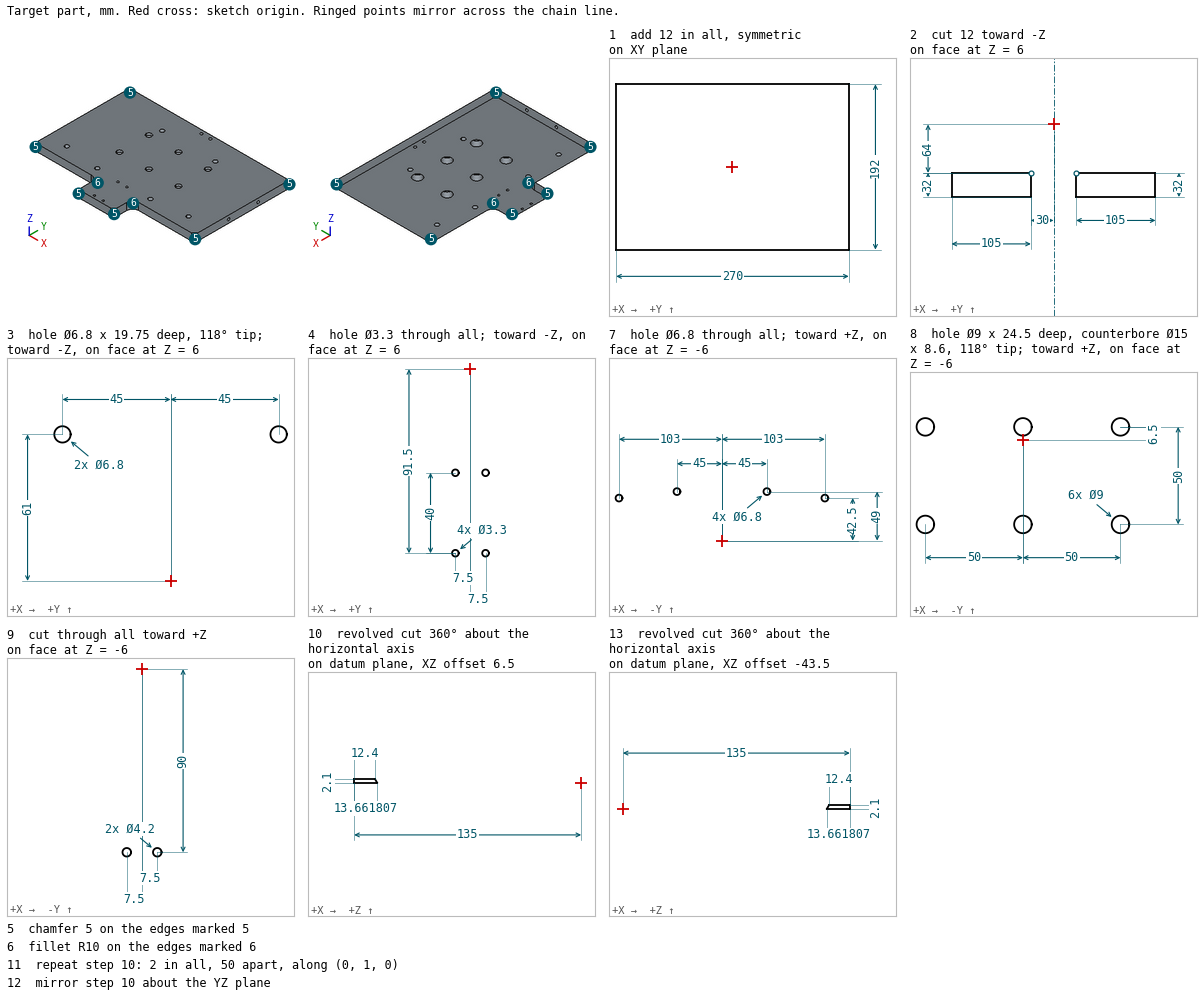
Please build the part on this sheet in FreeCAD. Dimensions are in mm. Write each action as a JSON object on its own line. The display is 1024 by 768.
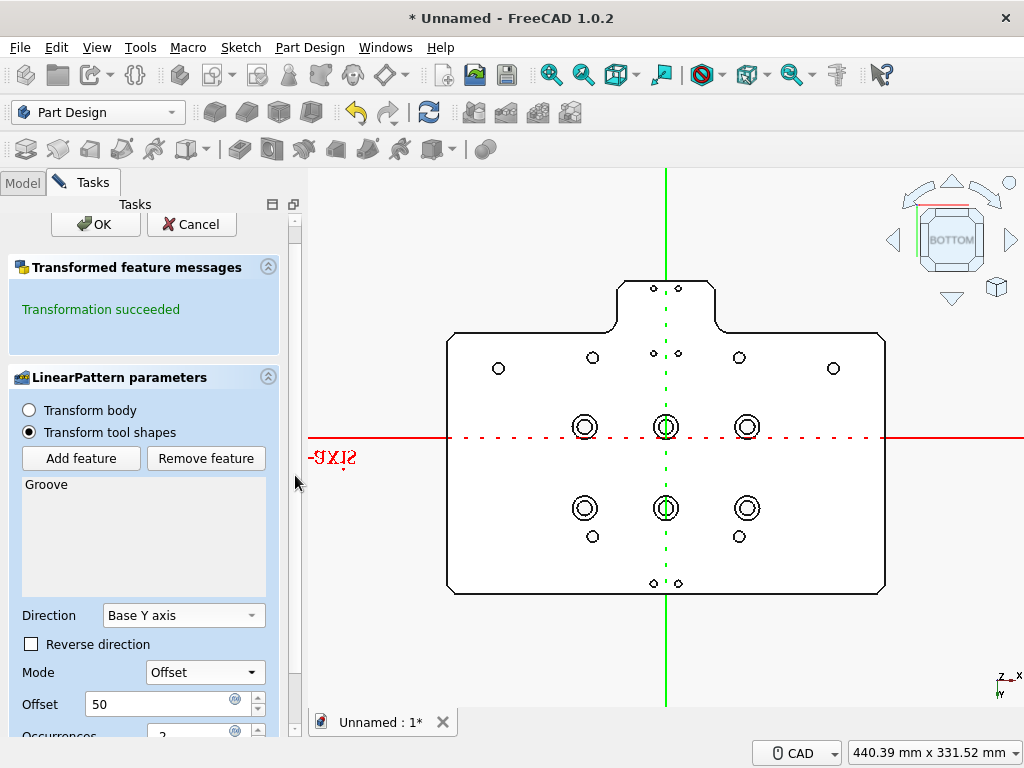
{"action": "left_click", "coordinate": [96, 243]}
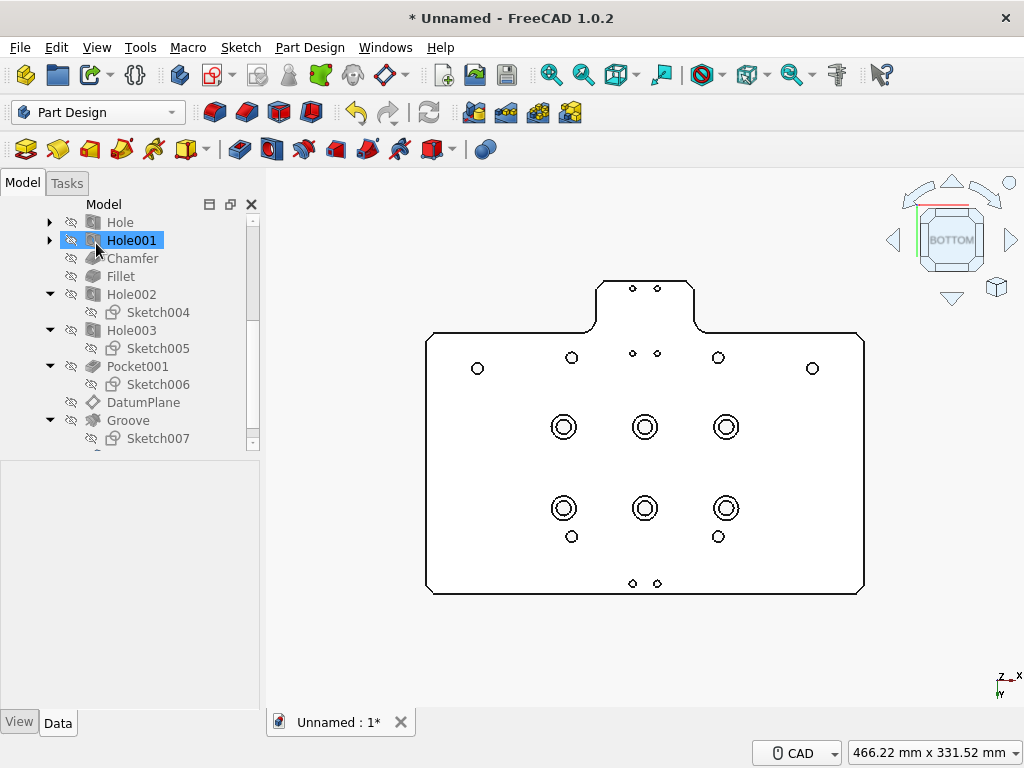
{"action": "left_click", "coordinate": [116, 420]}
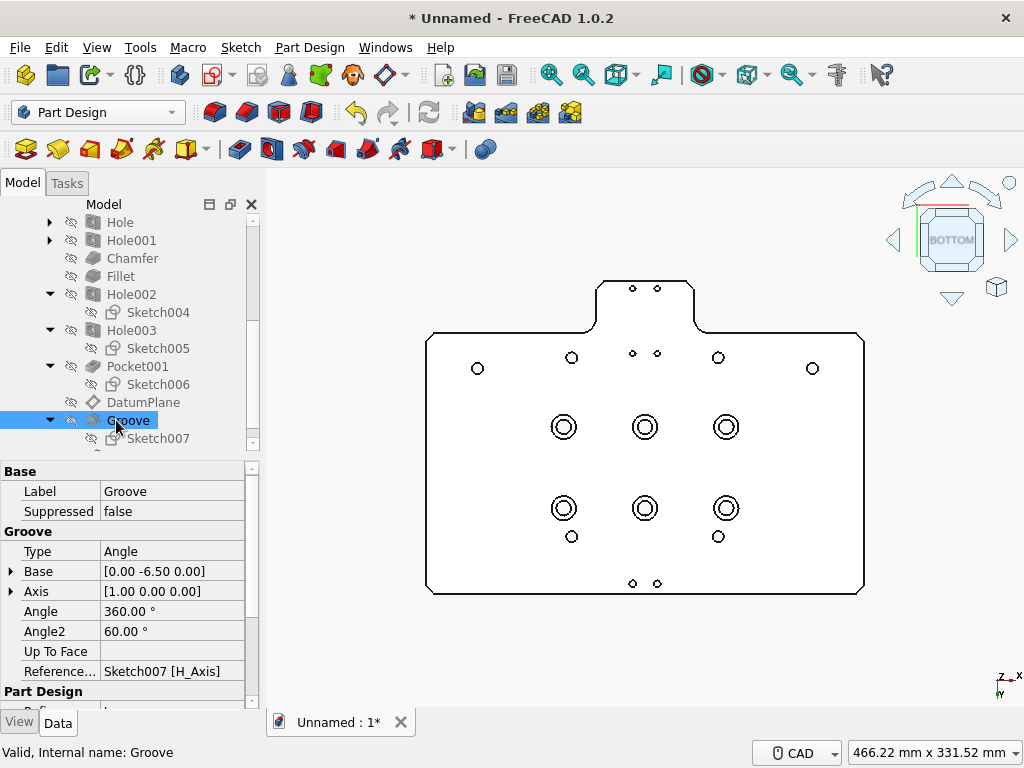
{"action": "left_click", "coordinate": [474, 112]}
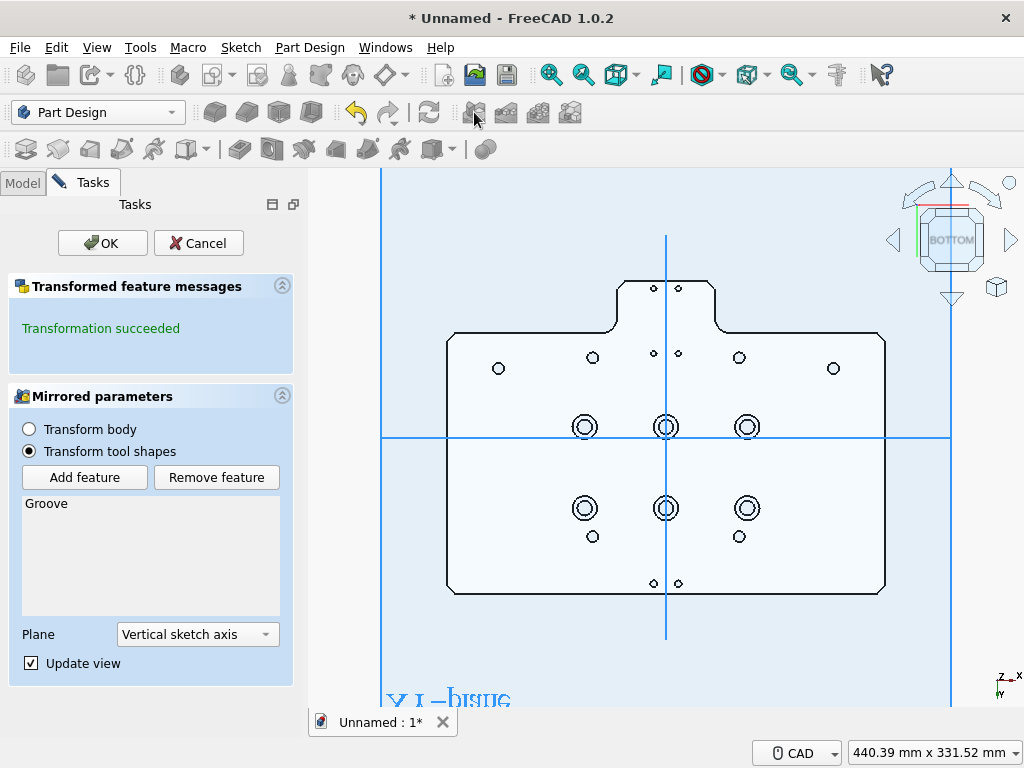
{"action": "left_click", "coordinate": [198, 634]}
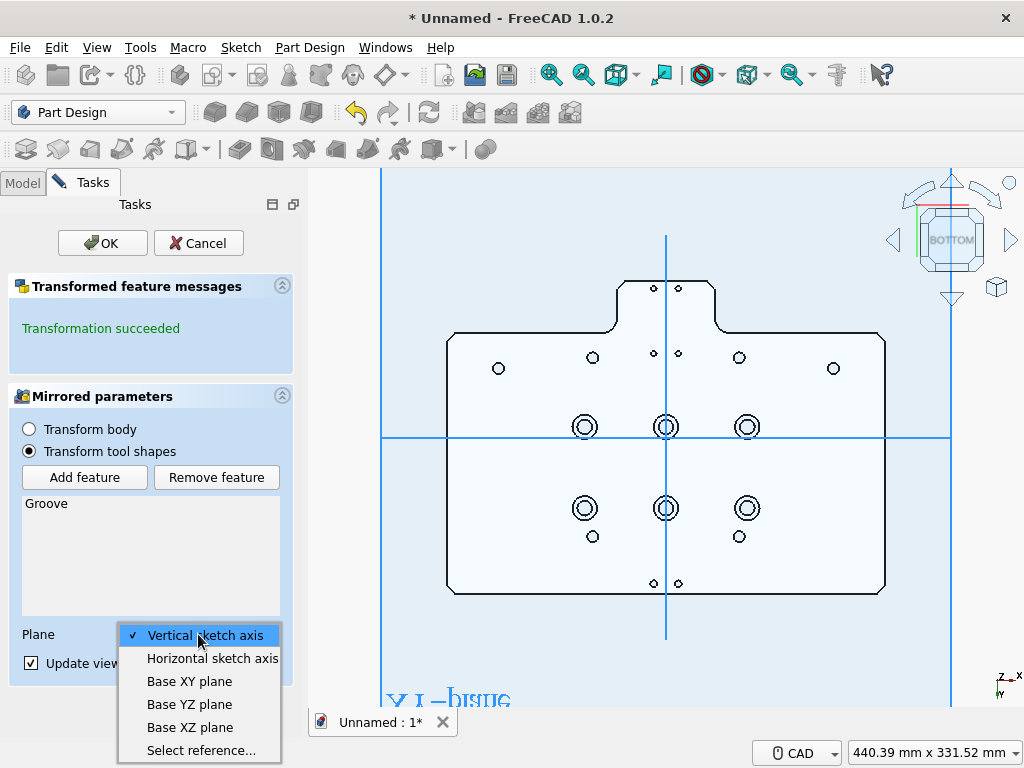
{"action": "left_click", "coordinate": [198, 704]}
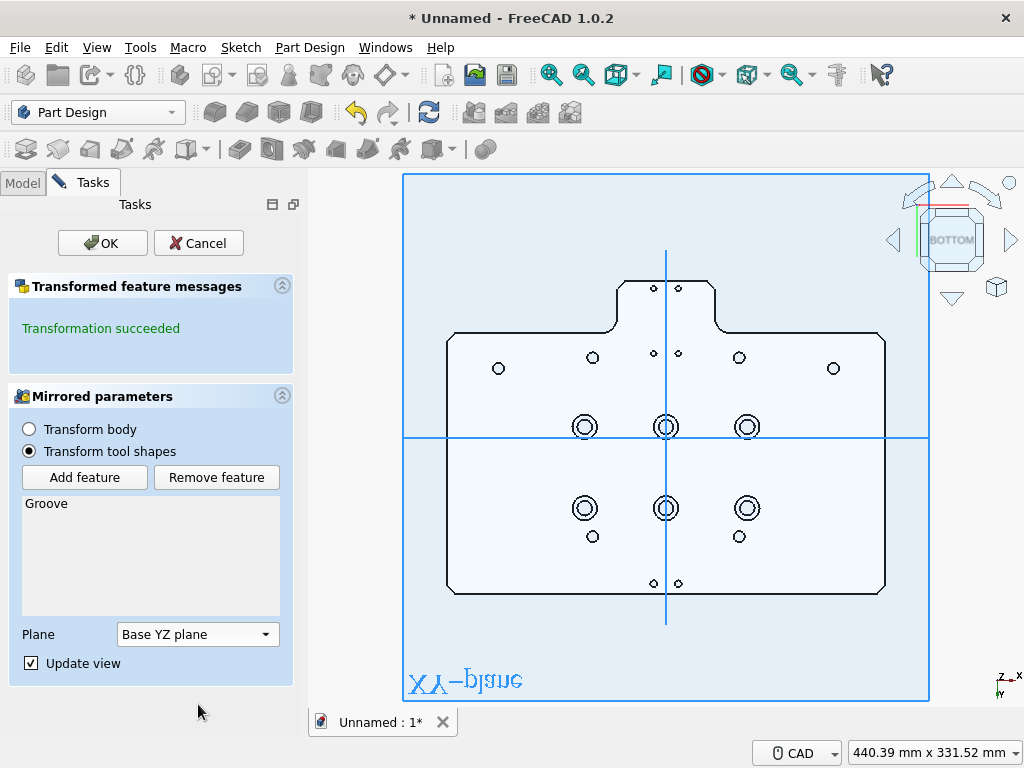
{"action": "left_click", "coordinate": [103, 243]}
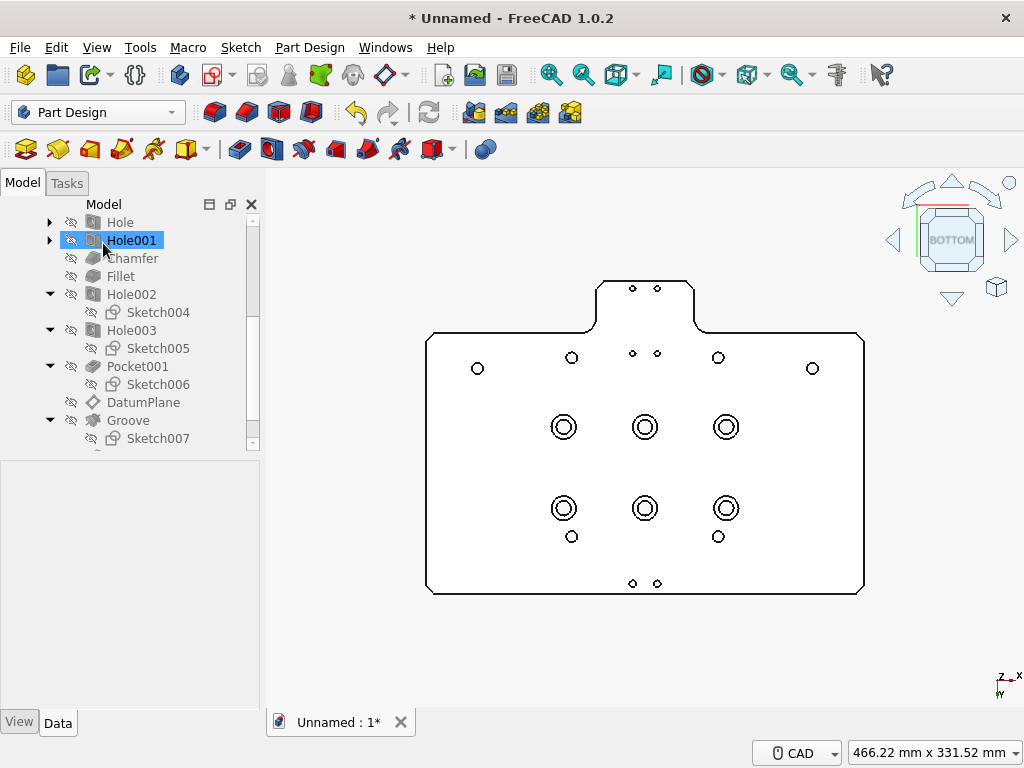
{"action": "scroll", "coordinate": [140, 326], "scroll_direction": "down", "scroll_amount": 3}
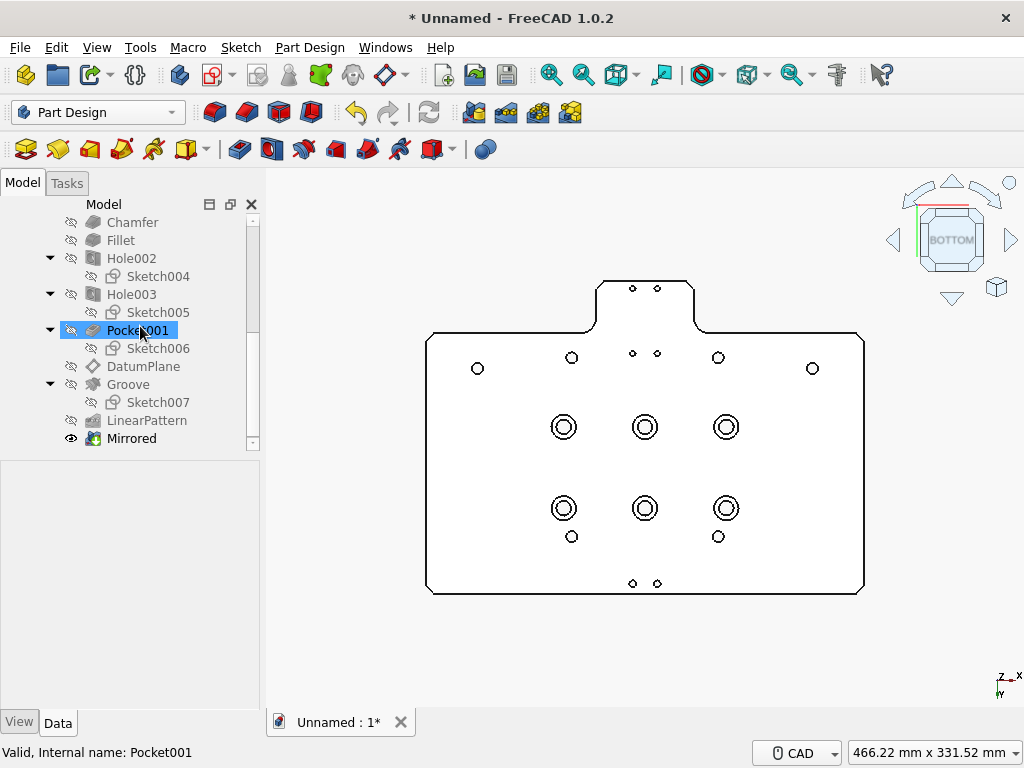
{"action": "scroll", "coordinate": [140, 326], "scroll_direction": "up", "scroll_amount": 15}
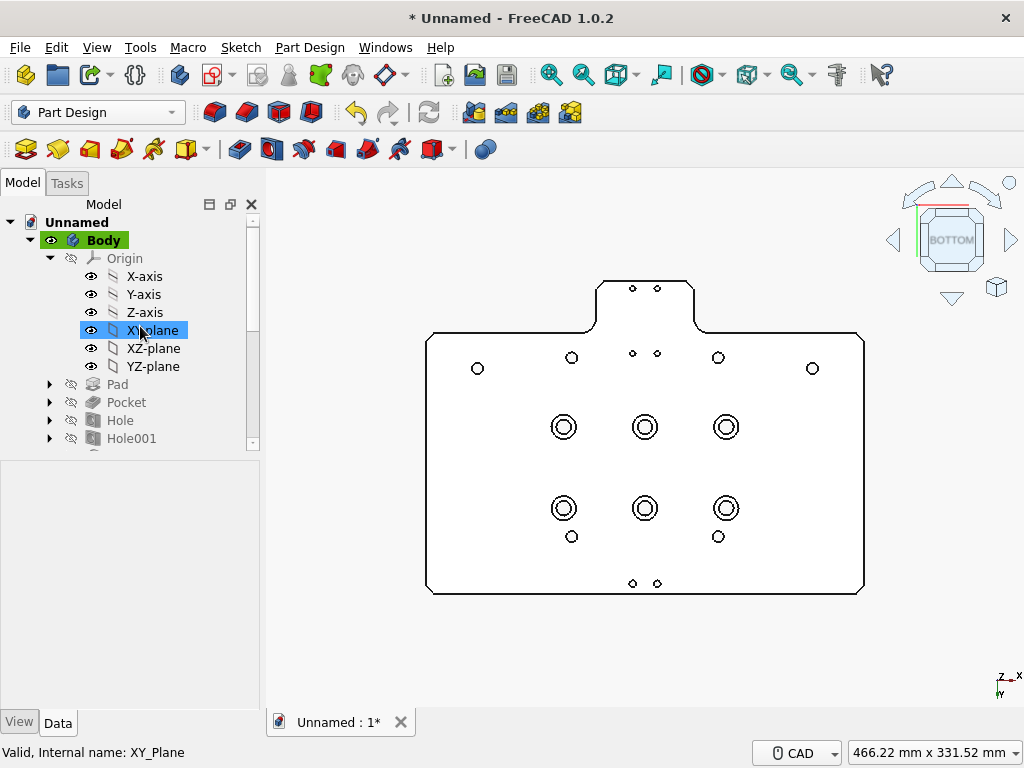
{"action": "left_click", "coordinate": [136, 348]}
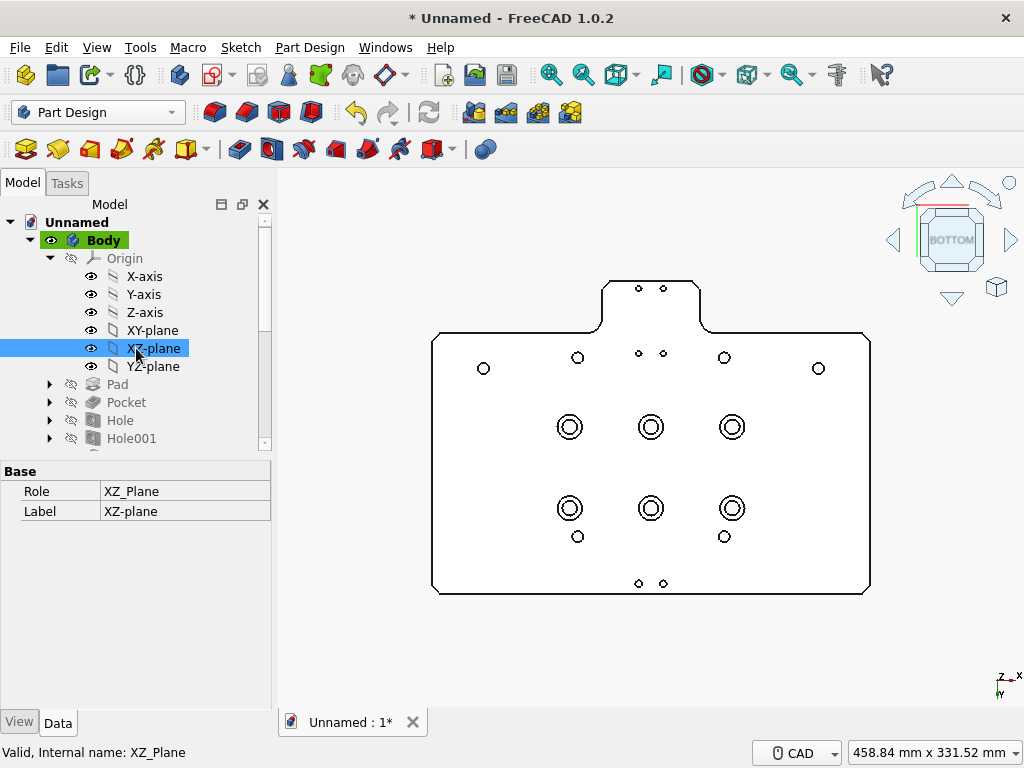
{"action": "left_click", "coordinate": [386, 76]}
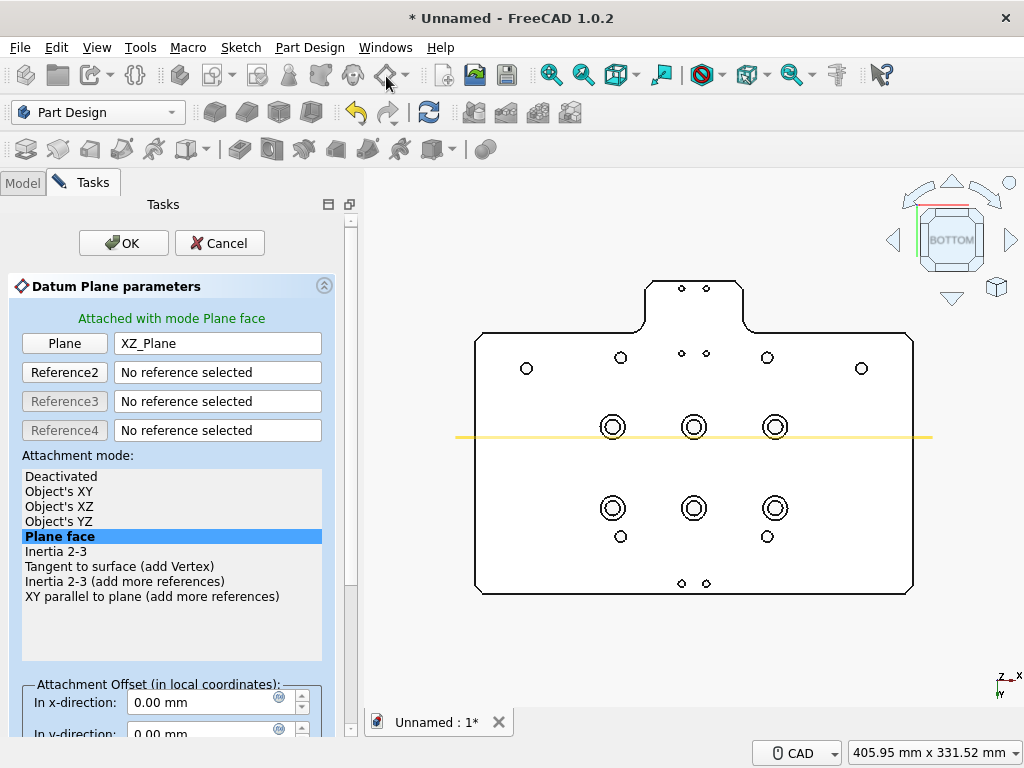
{"action": "scroll", "coordinate": [351, 475], "scroll_direction": "down", "scroll_amount": 2}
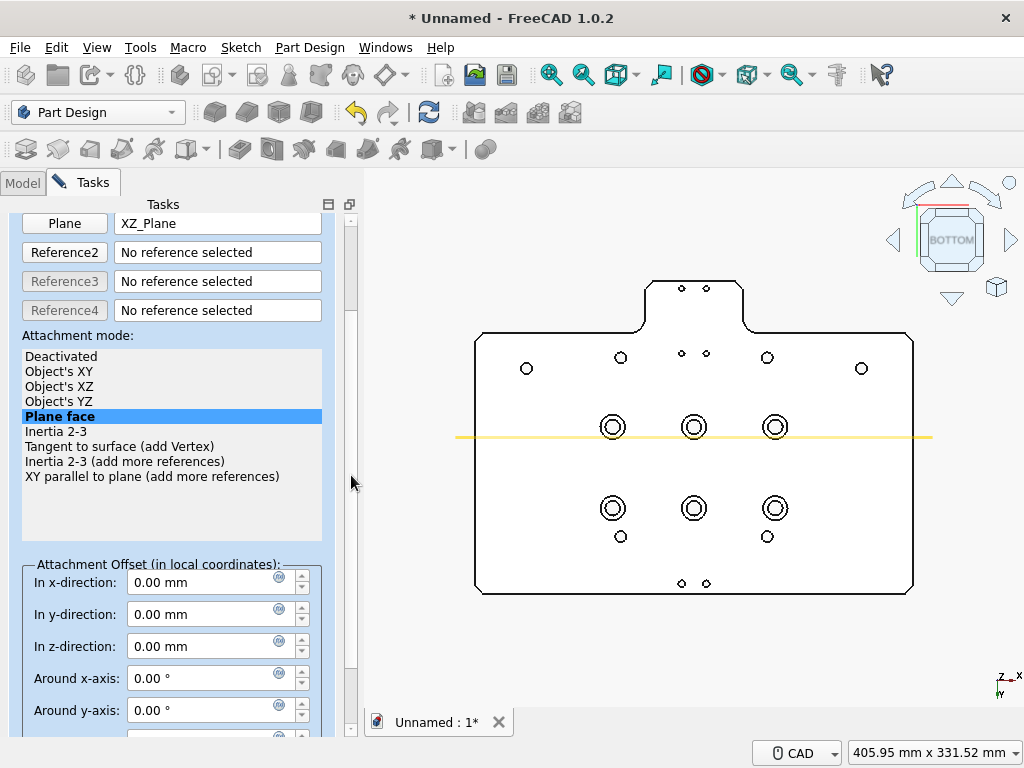
{"action": "triple_click", "coordinate": [210, 646]}